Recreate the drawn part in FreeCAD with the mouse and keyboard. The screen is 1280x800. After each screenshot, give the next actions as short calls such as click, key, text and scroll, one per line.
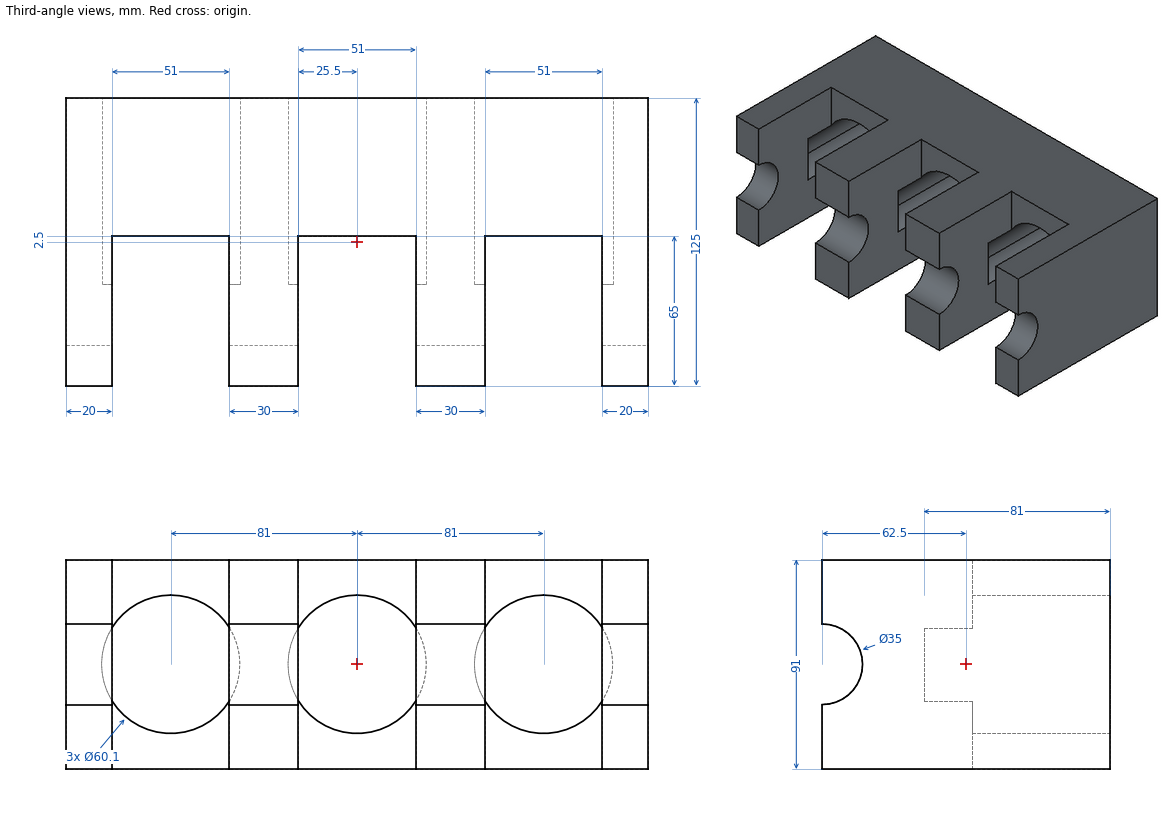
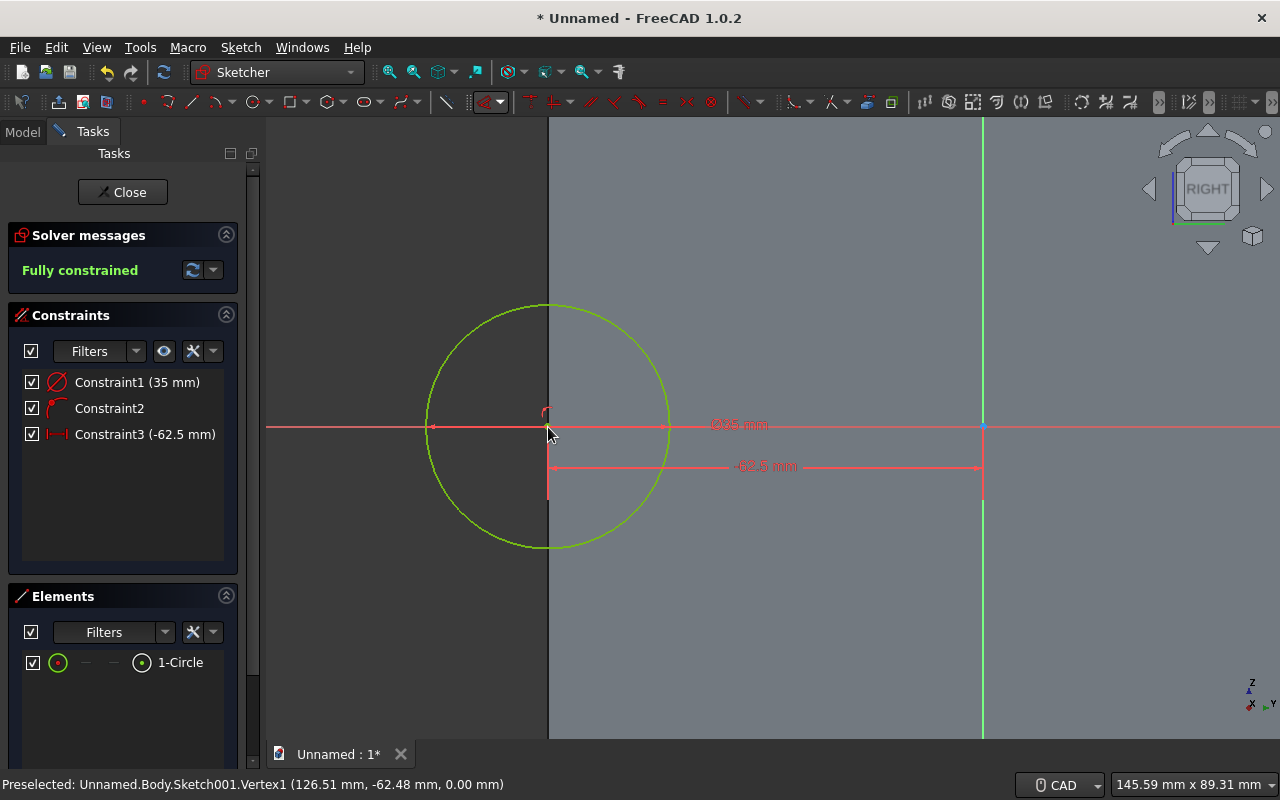
click(123, 192)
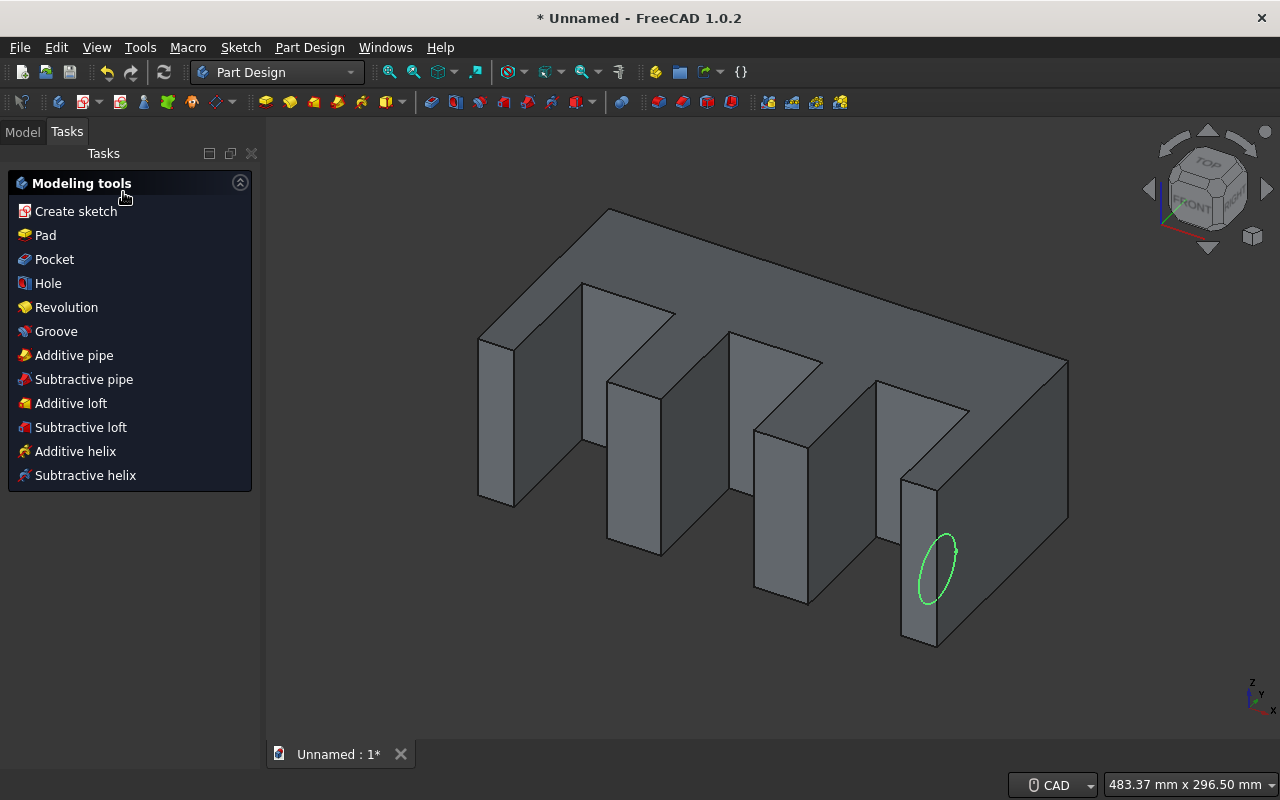
click(432, 102)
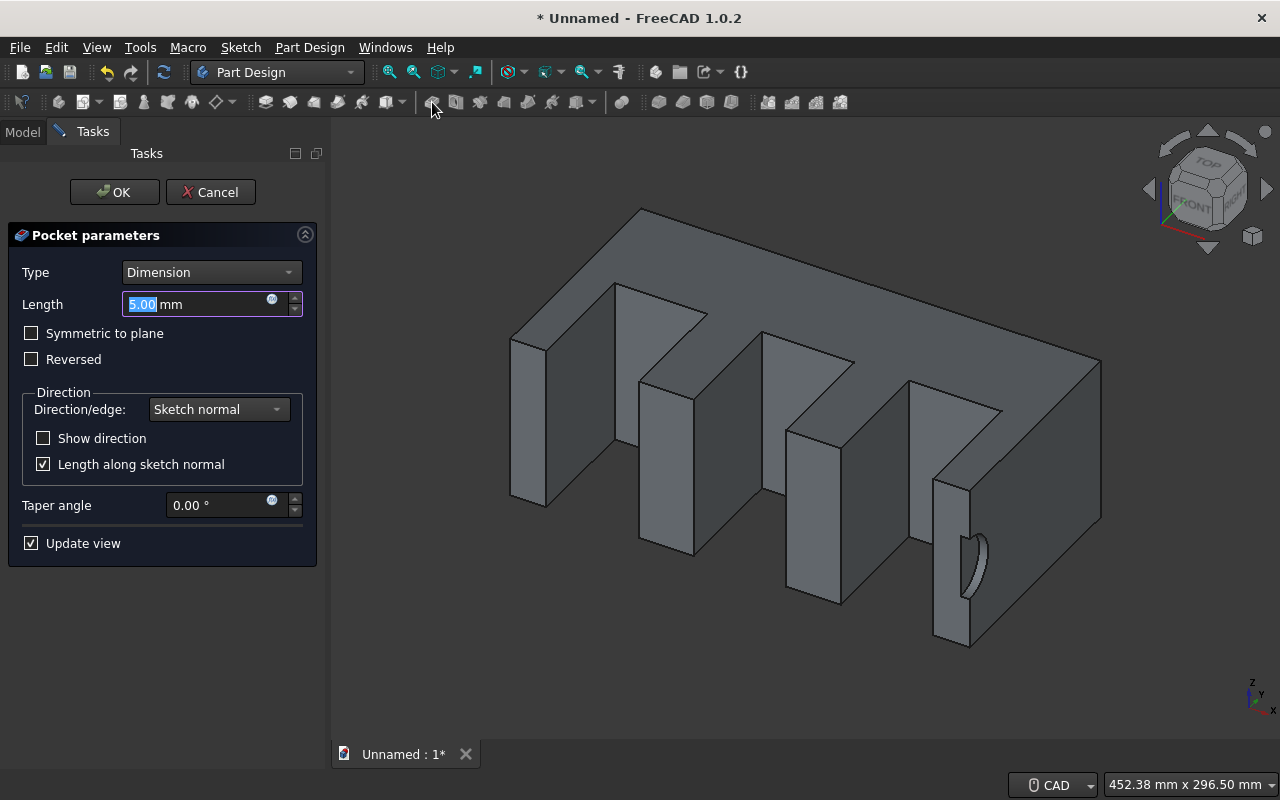
click(212, 272)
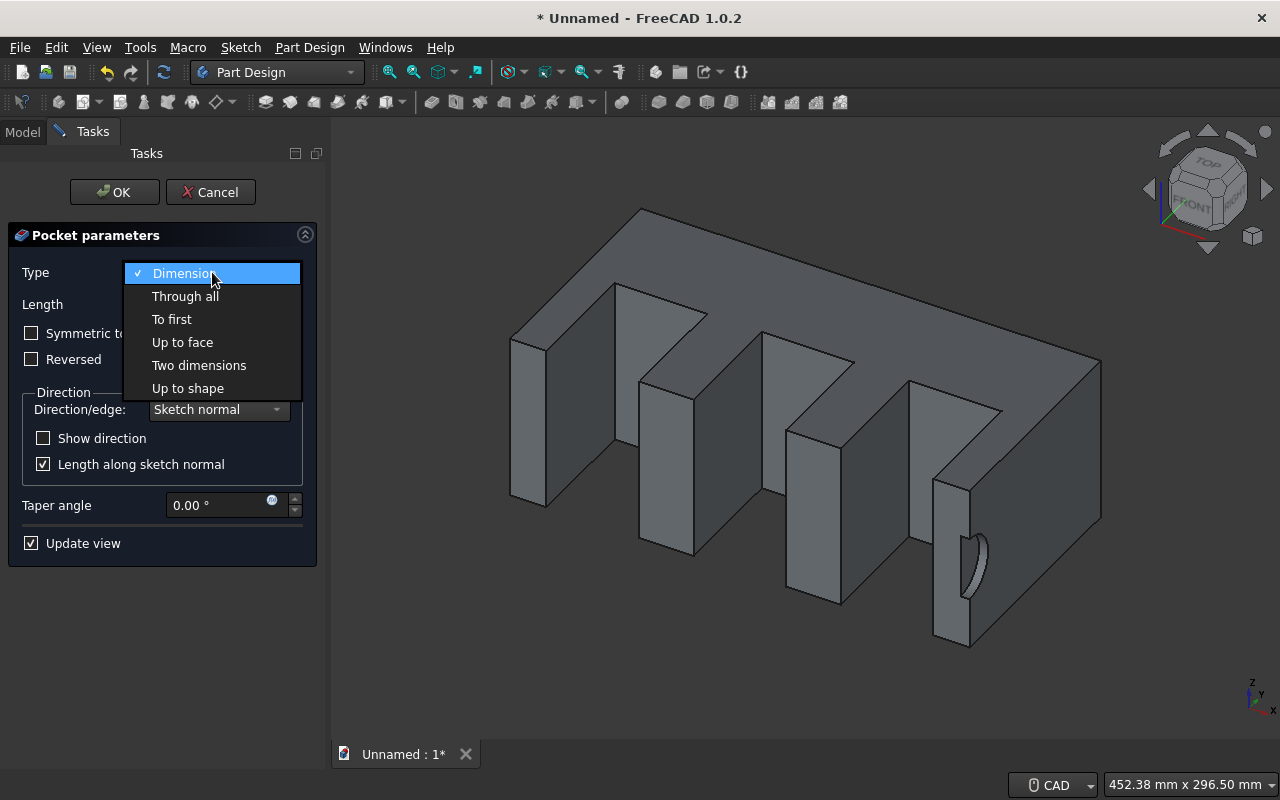
click(212, 296)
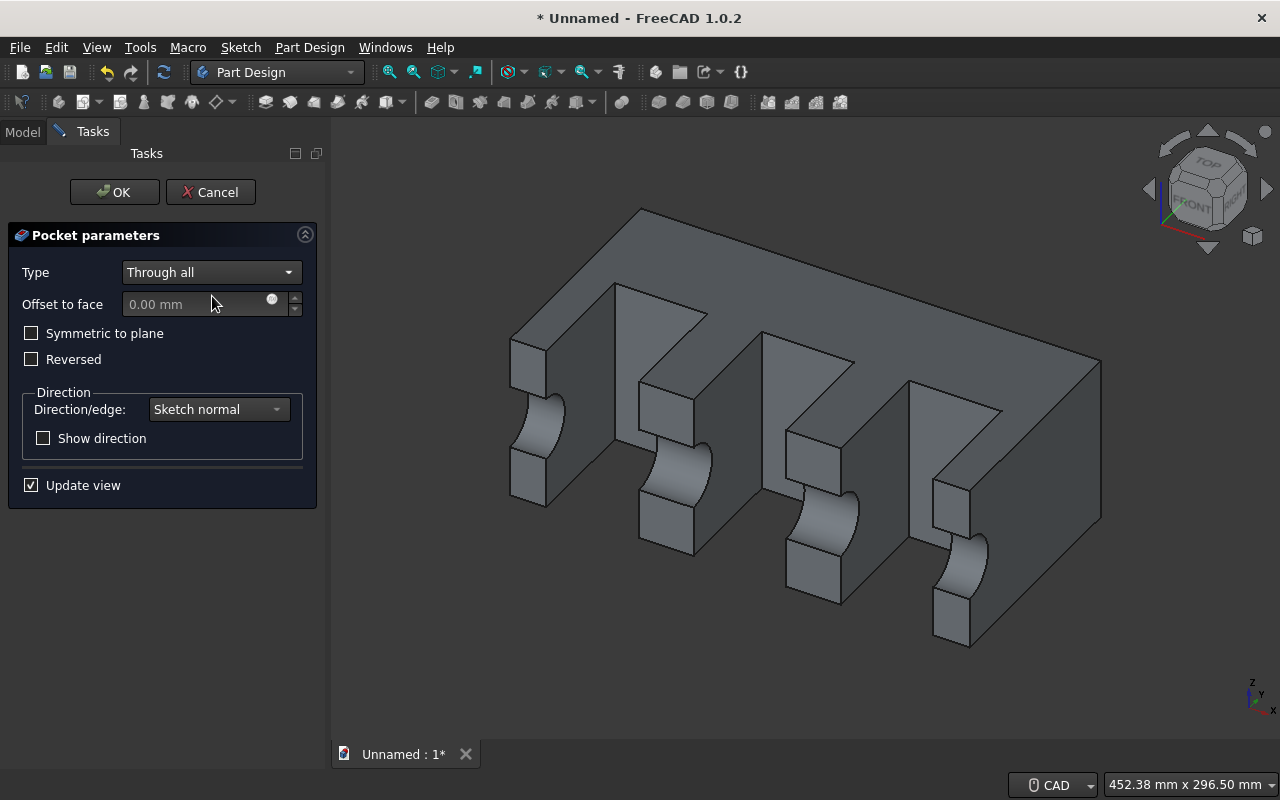
click(115, 192)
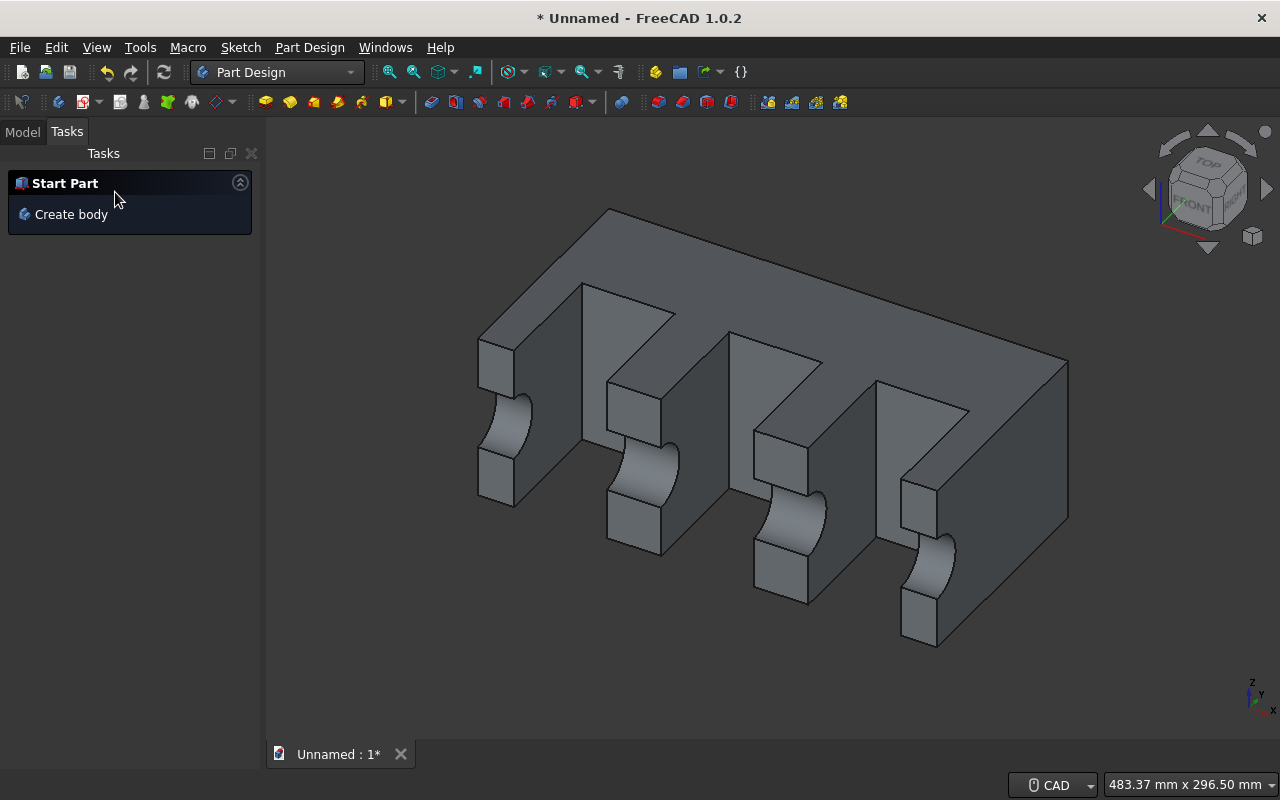
key(4)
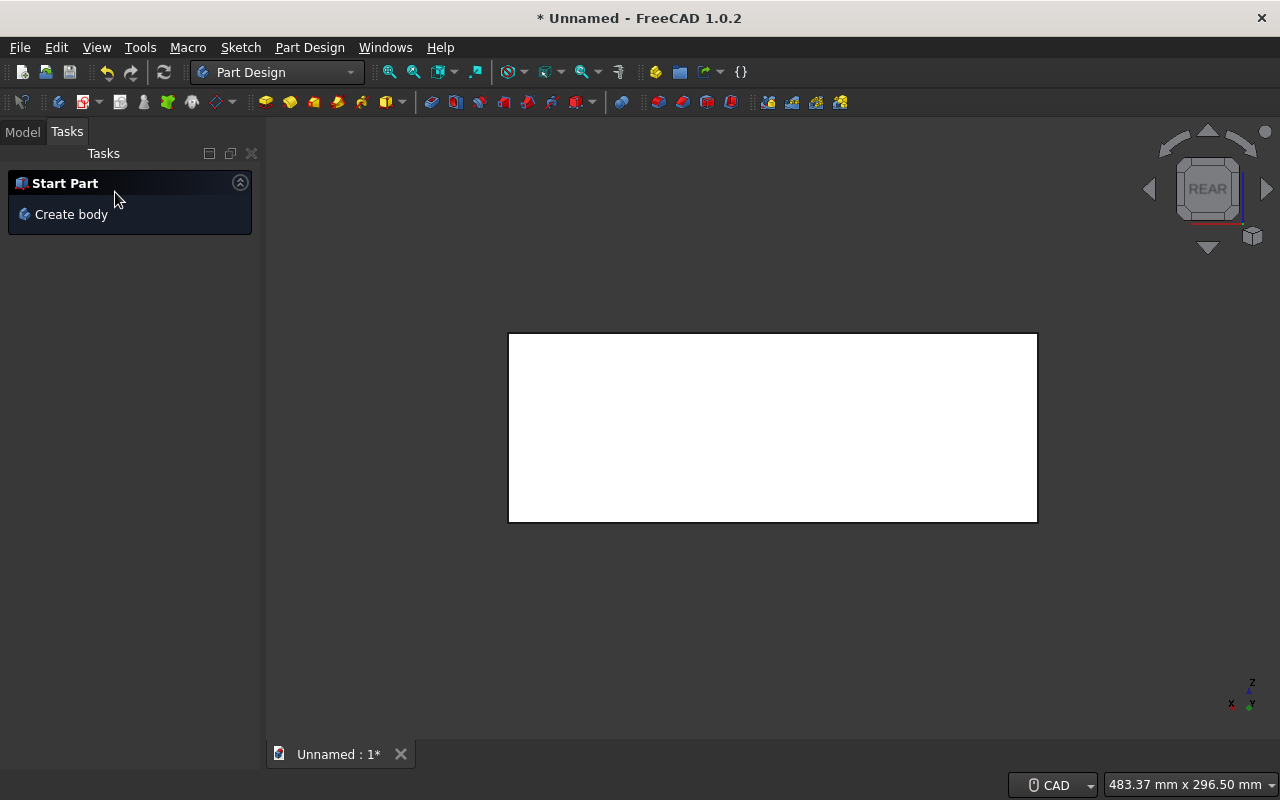
click(621, 427)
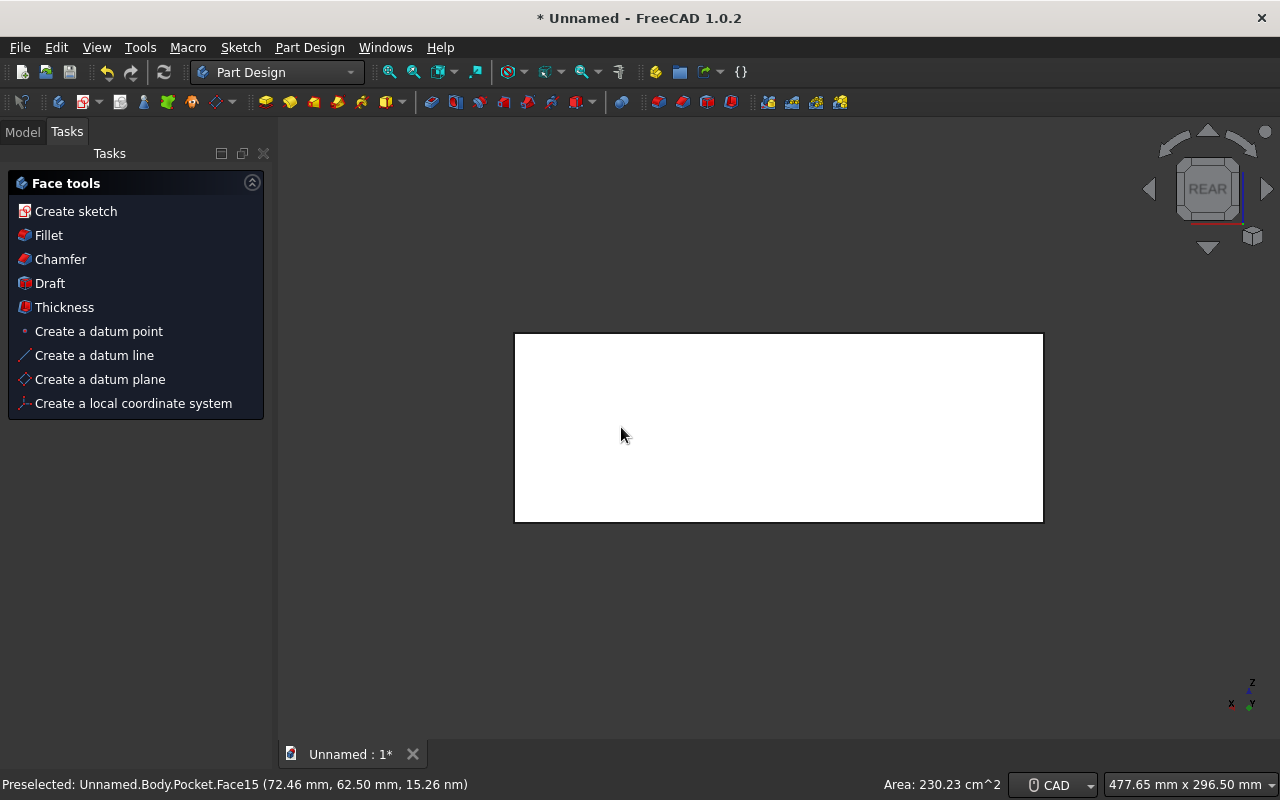
click(84, 102)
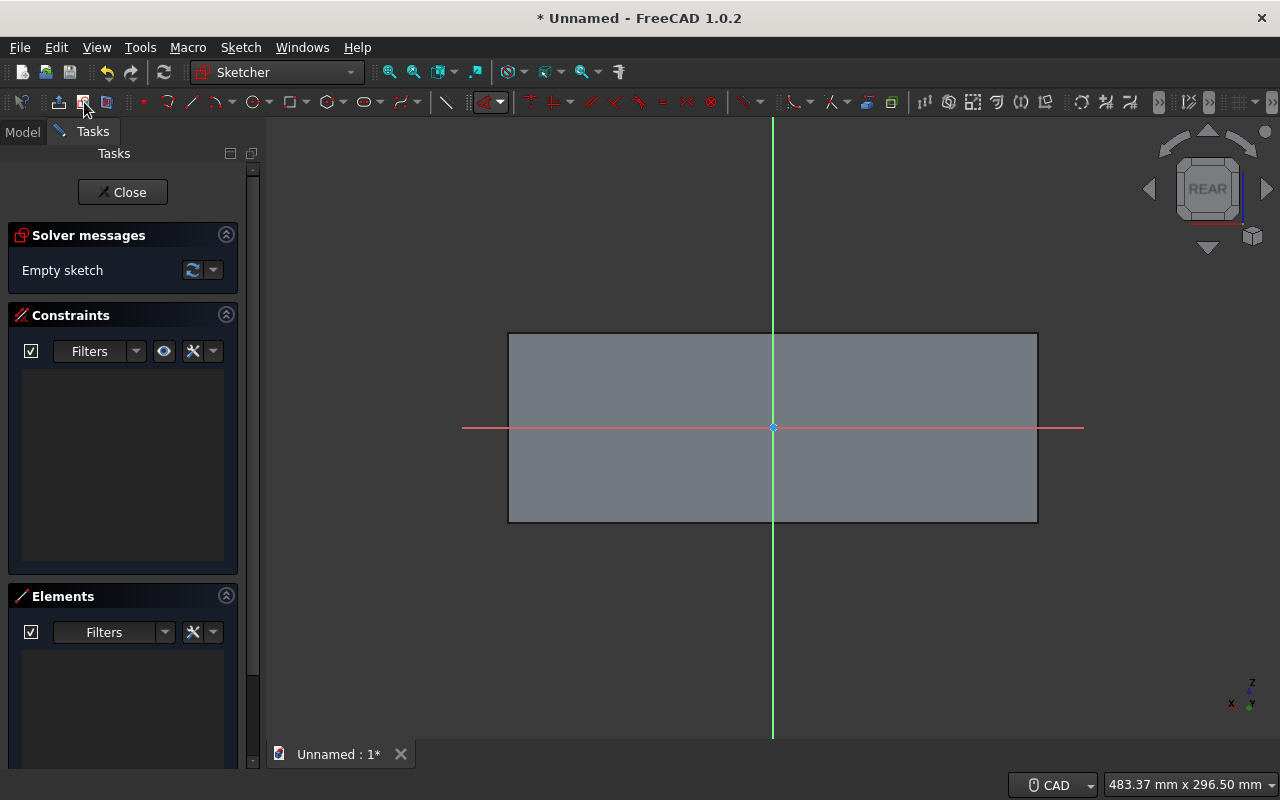
click(254, 102)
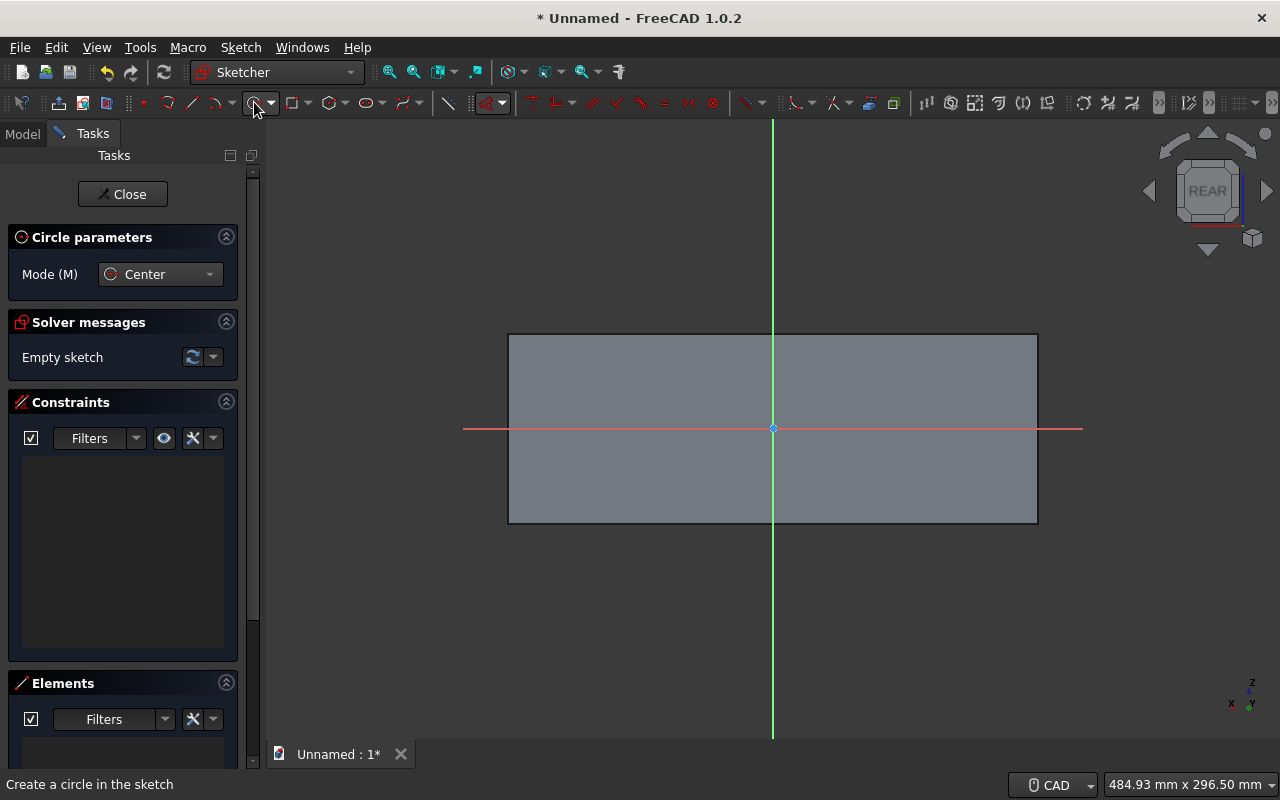
click(942, 429)
move(987, 385)